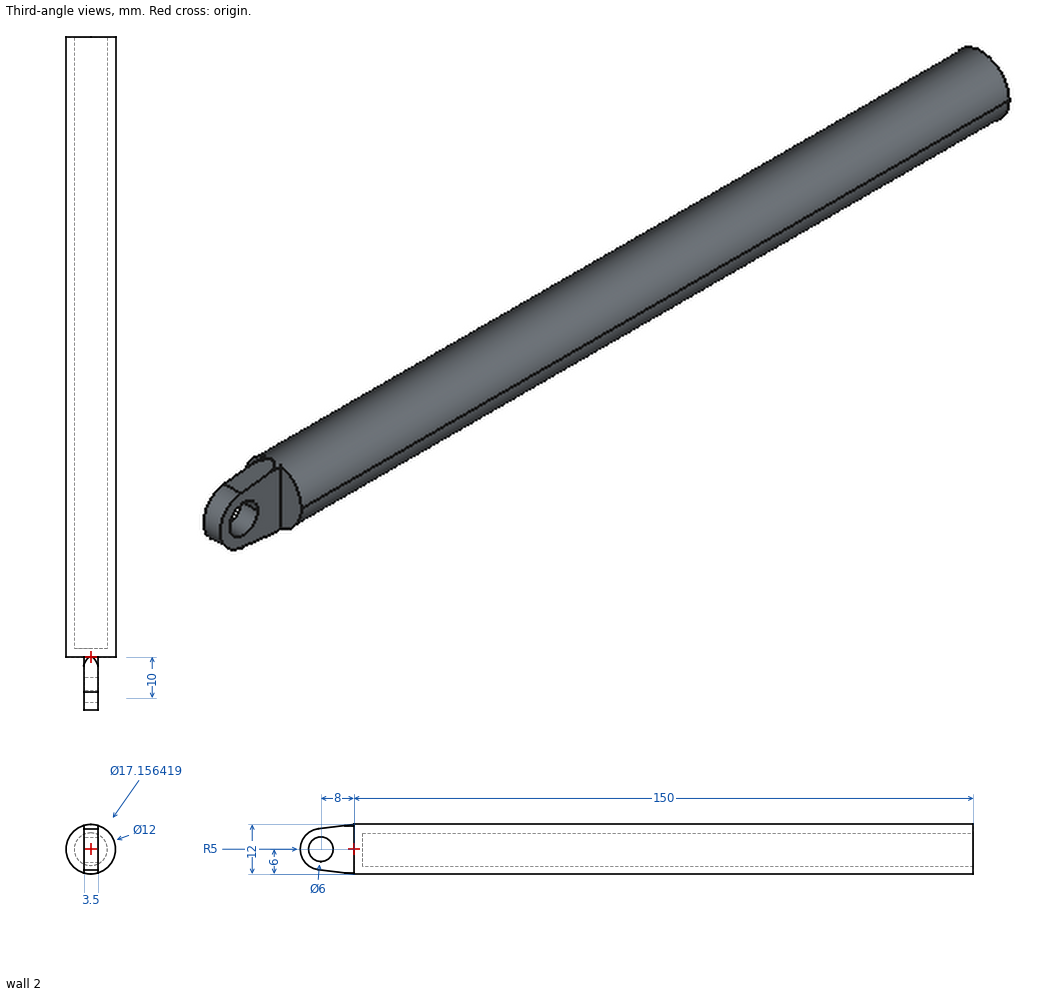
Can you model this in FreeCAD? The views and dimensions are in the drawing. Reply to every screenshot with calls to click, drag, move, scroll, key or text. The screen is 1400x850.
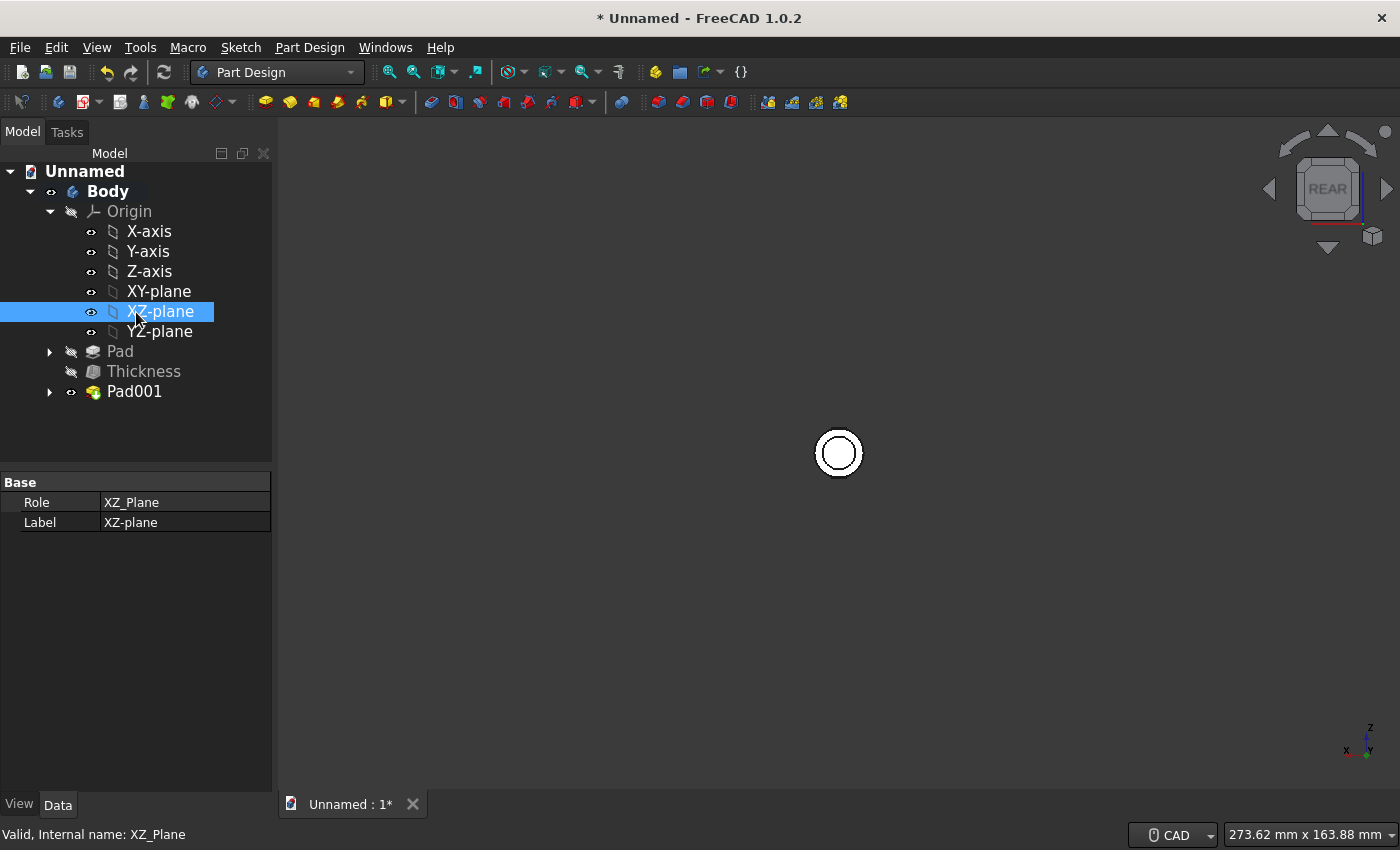
click(216, 102)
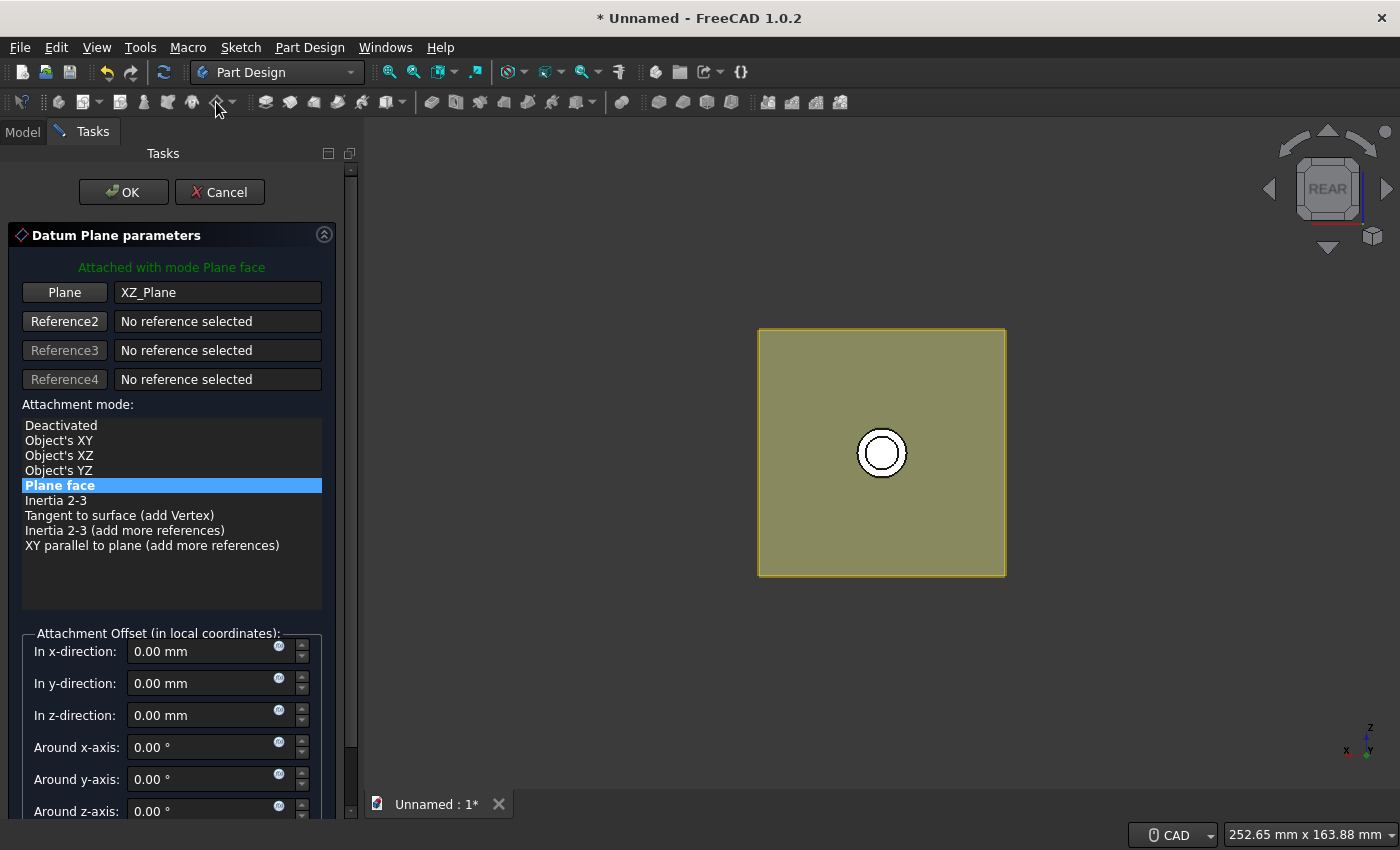
triple_click(210, 715)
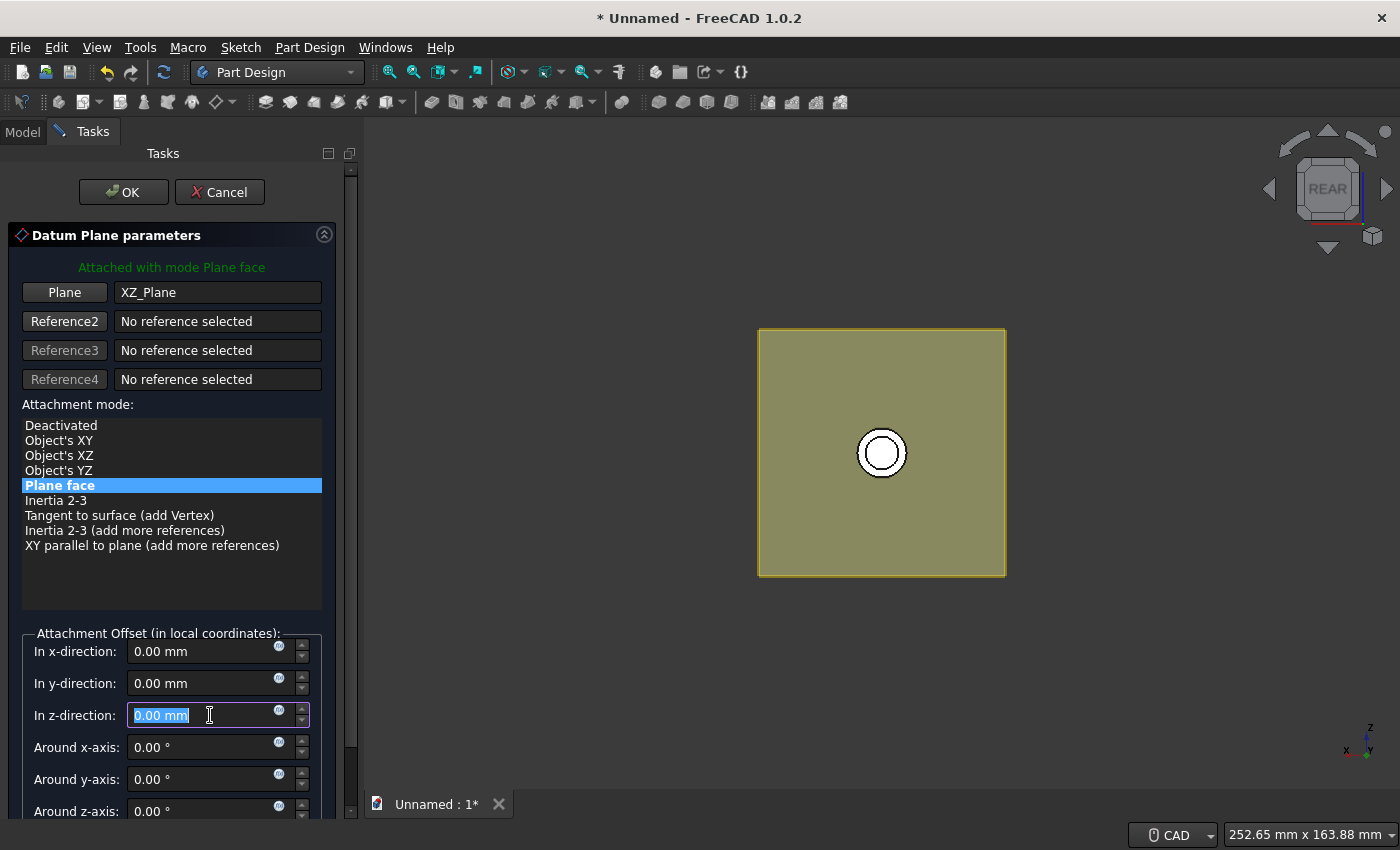
text(10)
key(Tab)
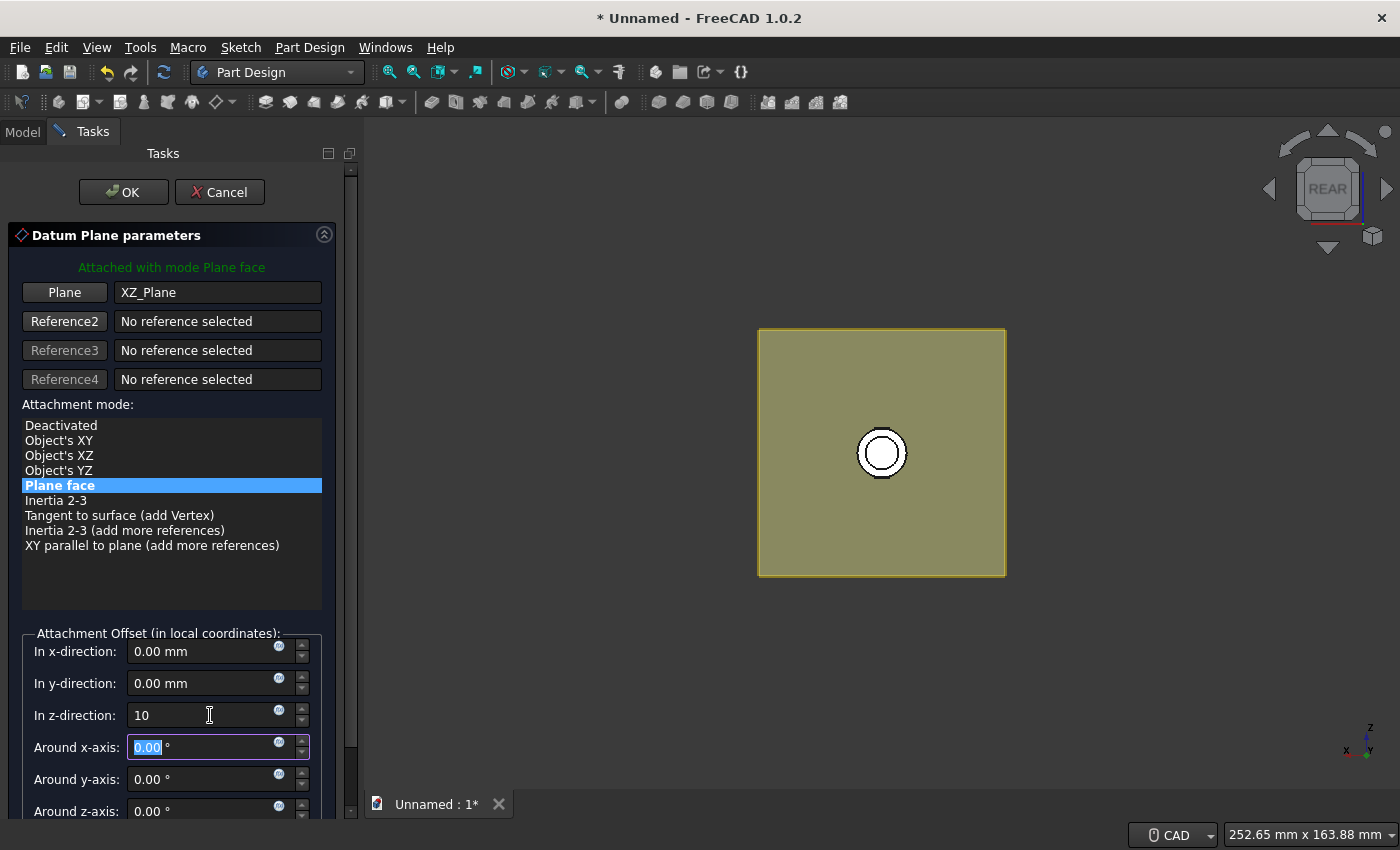
click(124, 192)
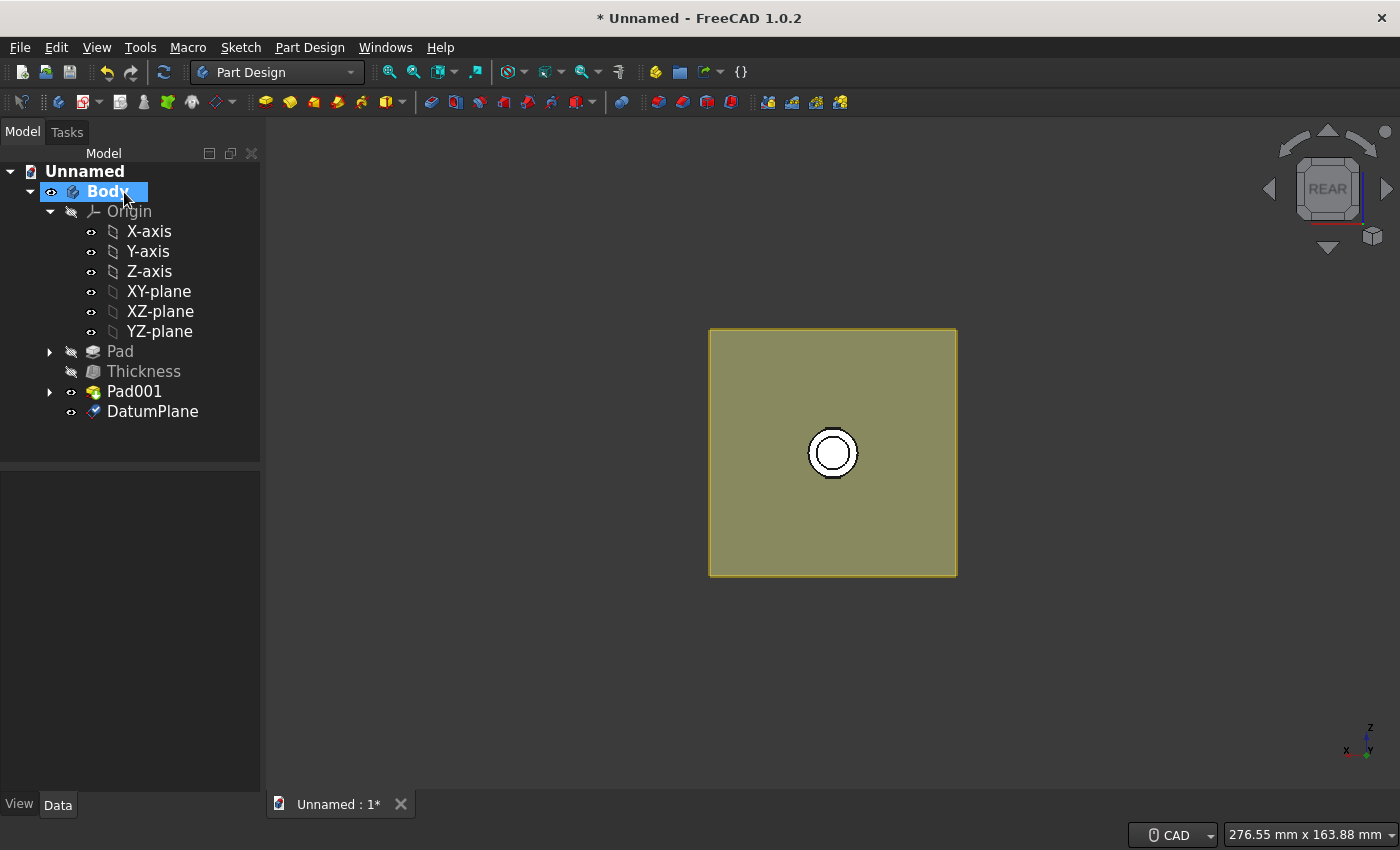
click(116, 412)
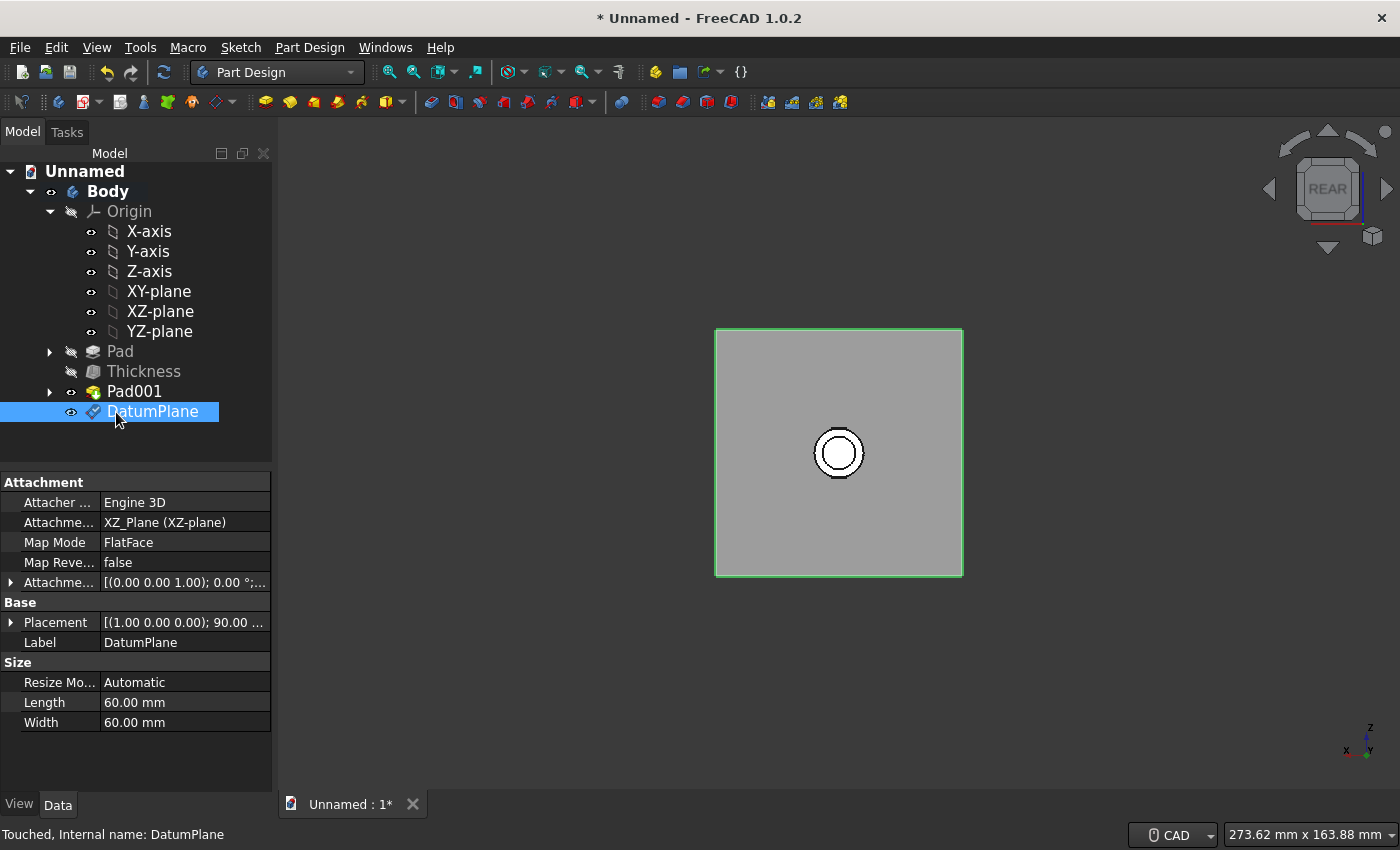
click(84, 102)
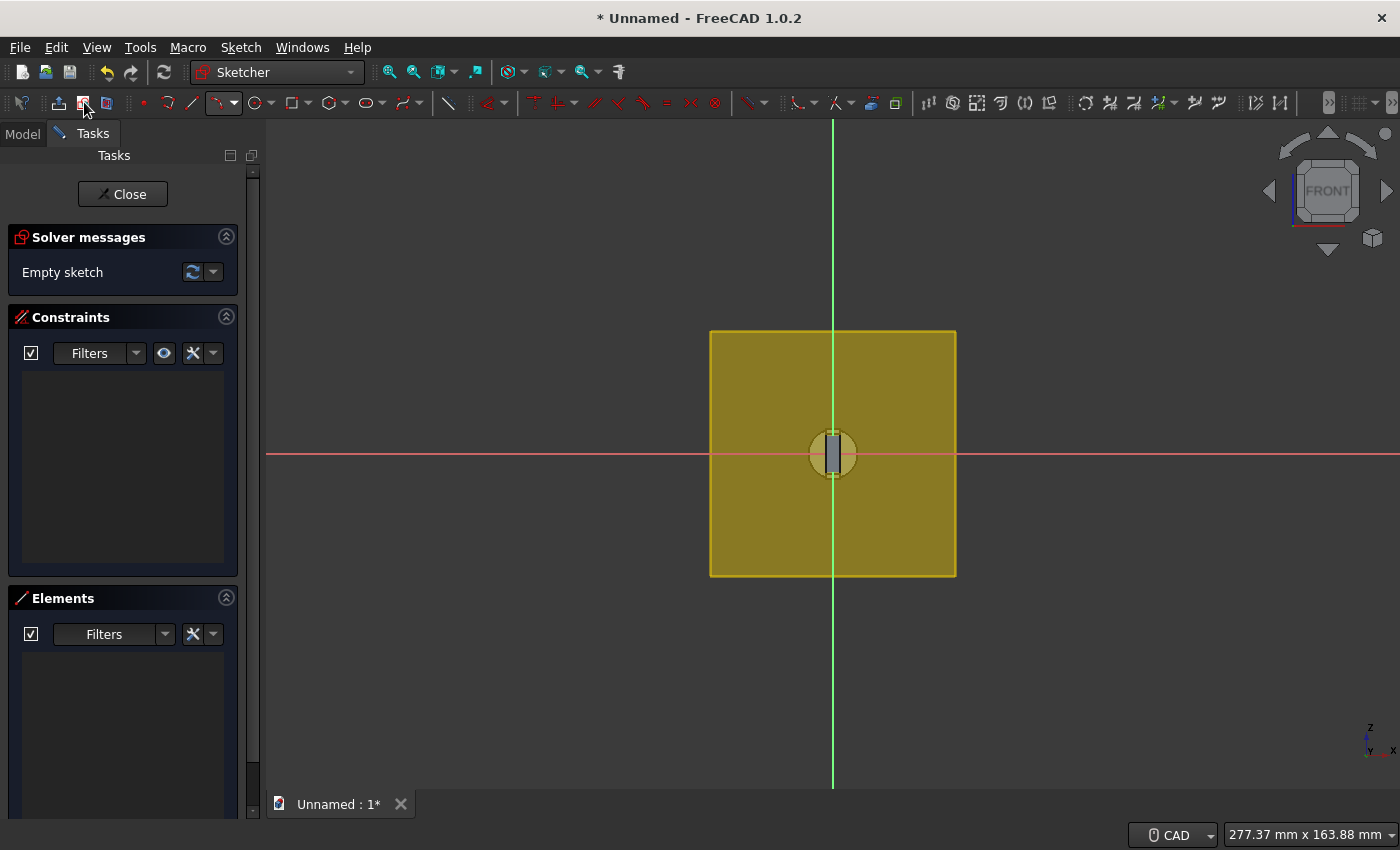
click(108, 104)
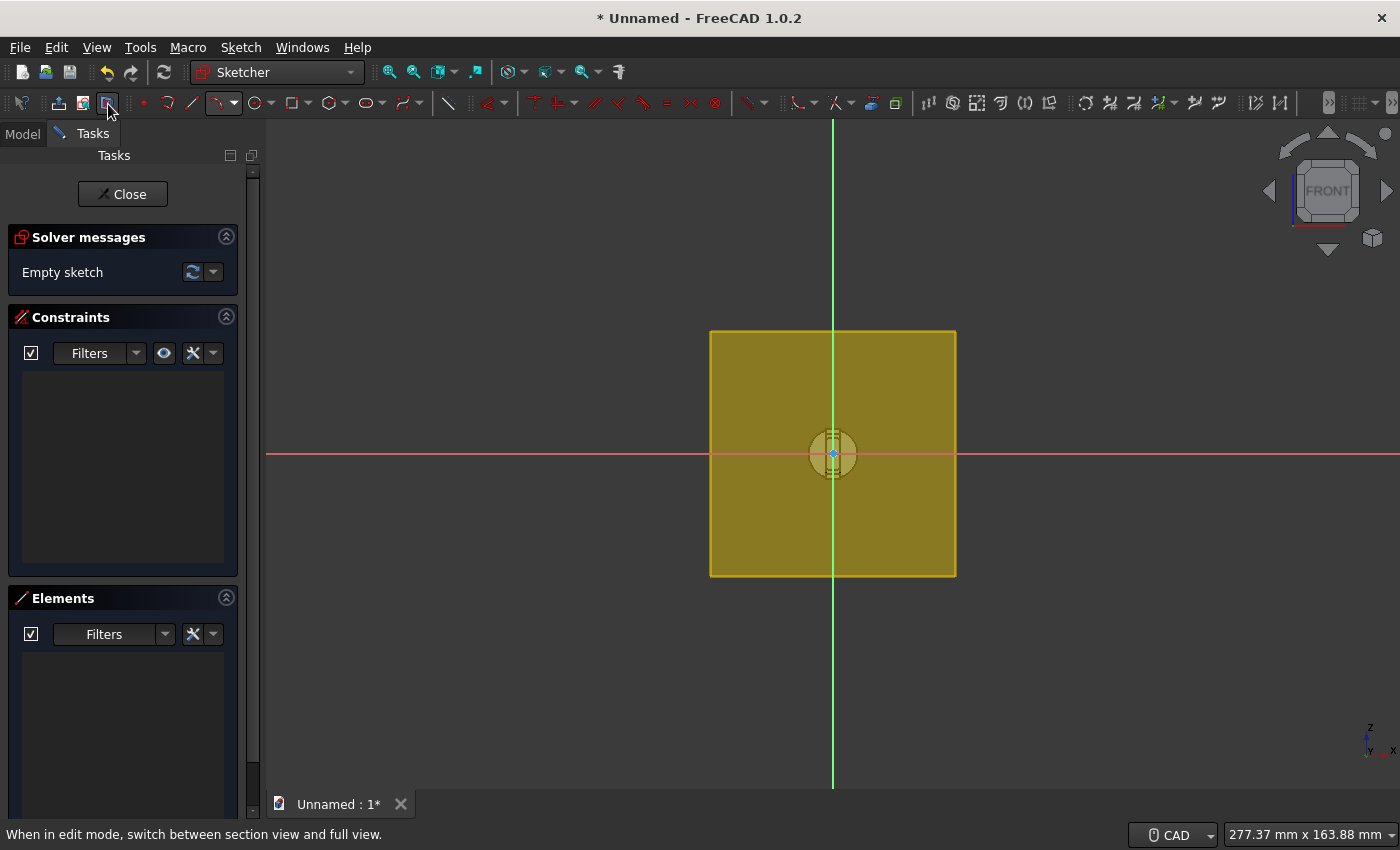
scroll(847, 454, up, 9)